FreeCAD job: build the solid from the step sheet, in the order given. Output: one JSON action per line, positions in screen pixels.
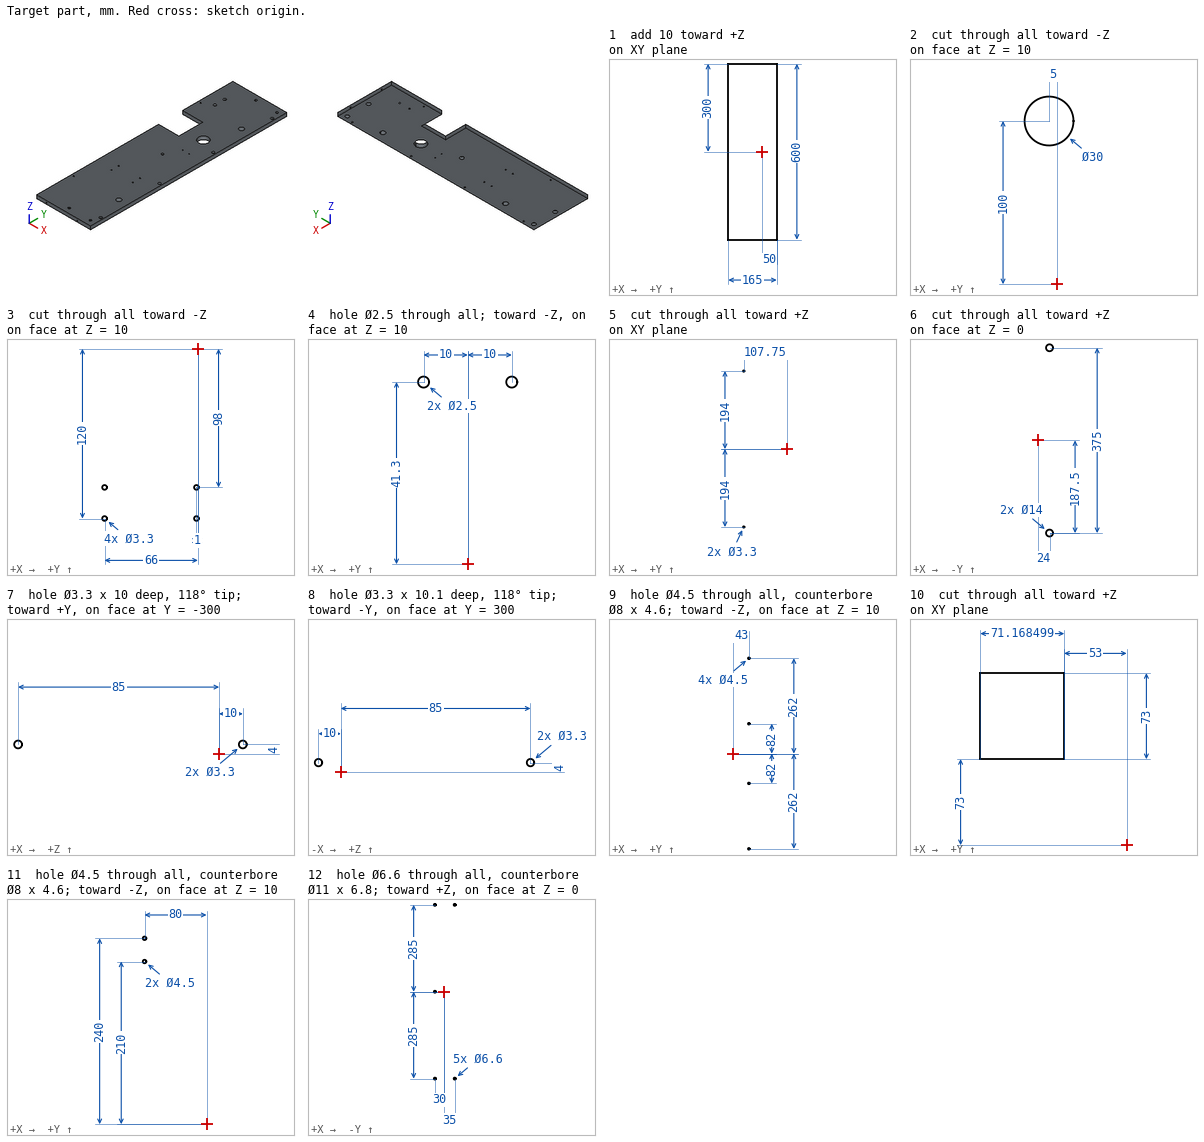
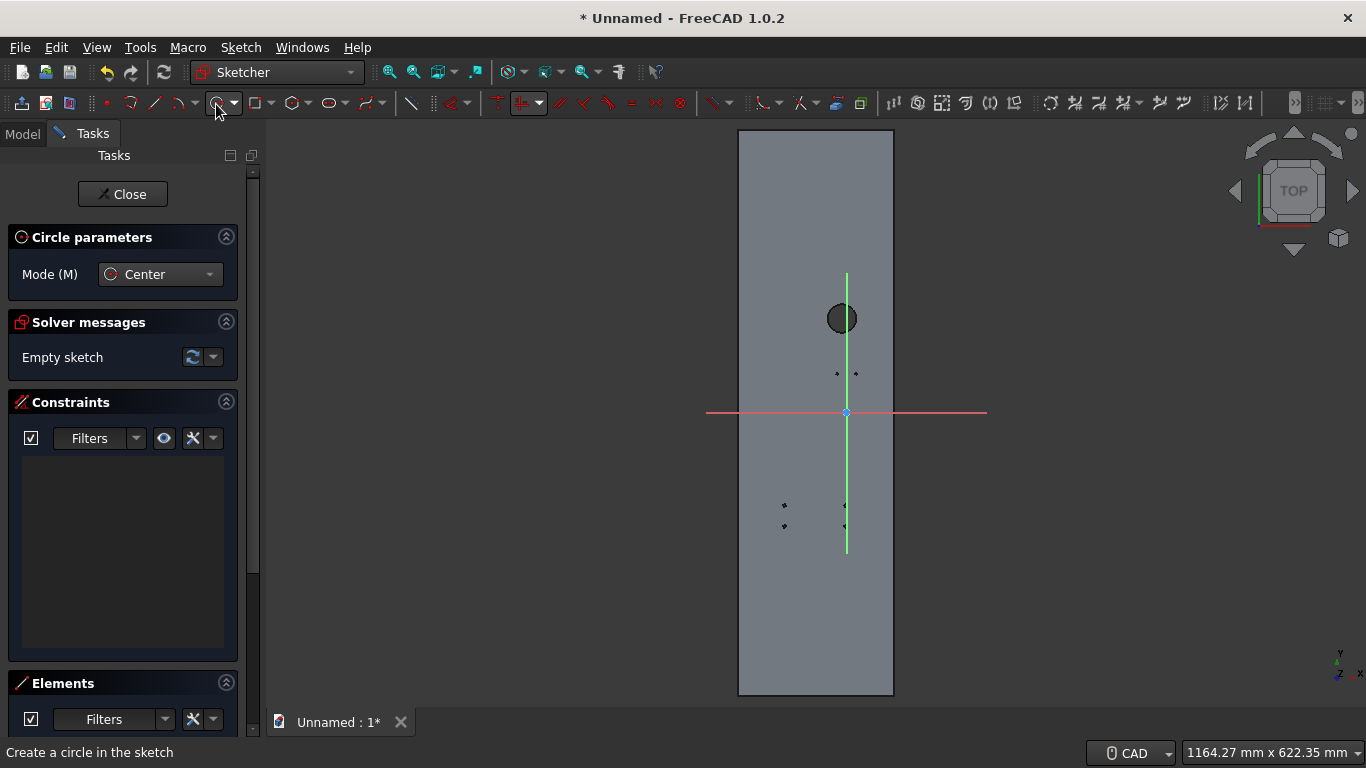
{"action": "scroll", "coordinate": [745, 230], "scroll_direction": "up", "scroll_amount": 14}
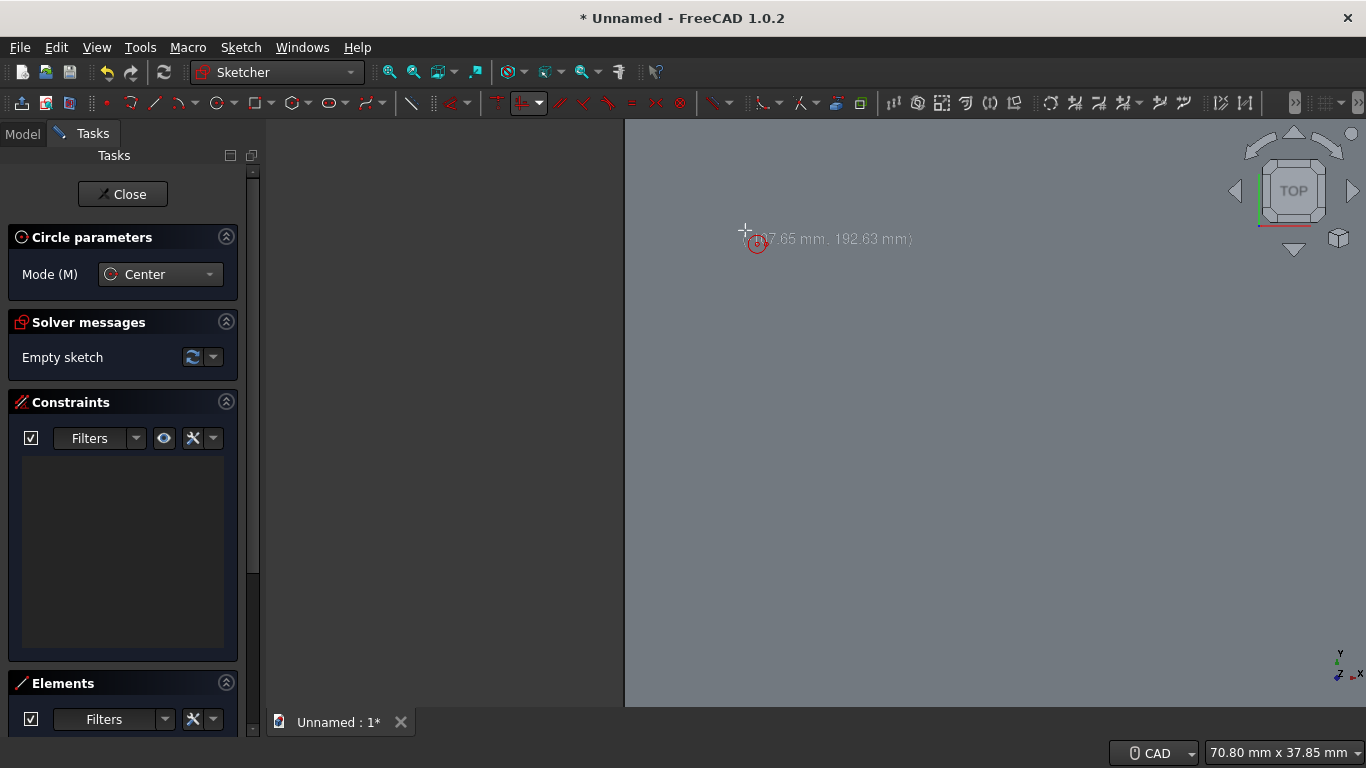
{"action": "scroll", "coordinate": [695, 230], "scroll_direction": "down", "scroll_amount": 14}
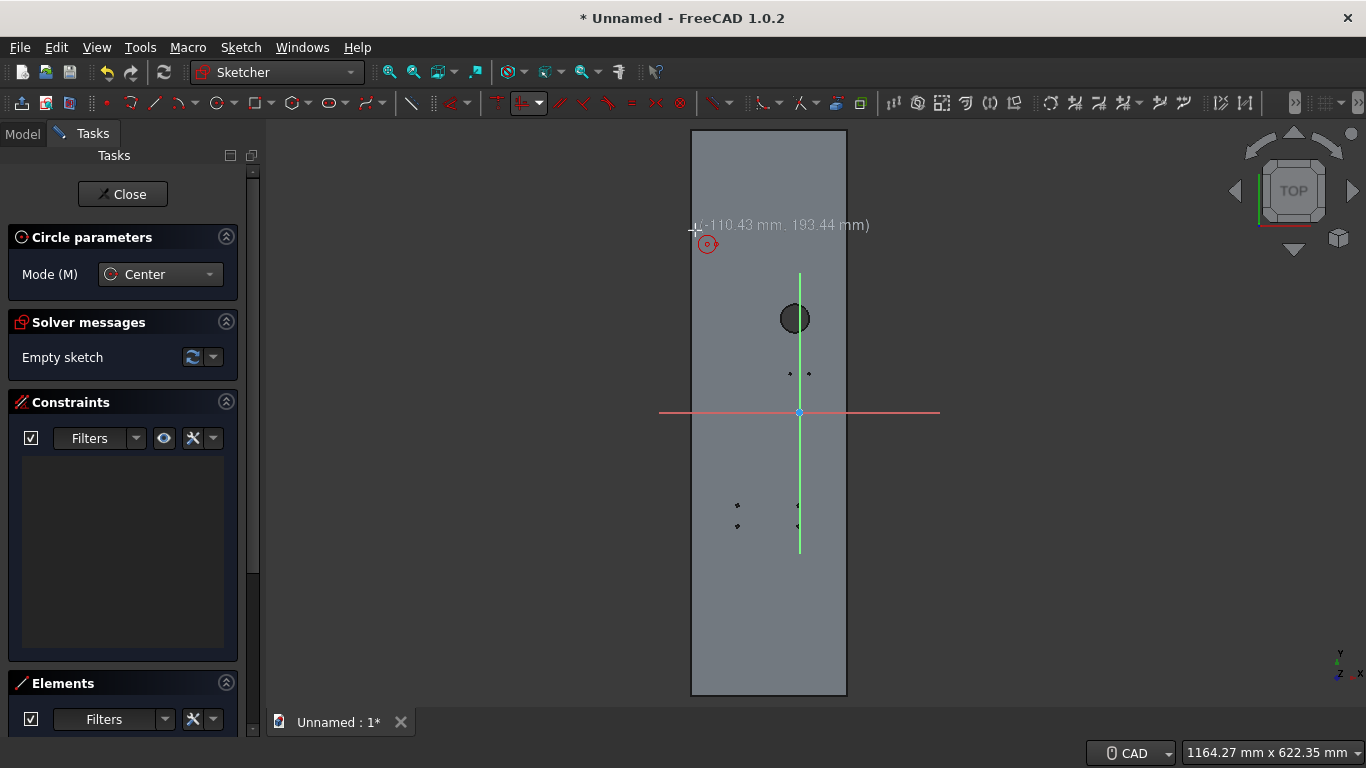
{"action": "left_click", "coordinate": [698, 230]}
{"action": "mouse_move", "coordinate": [699, 229]}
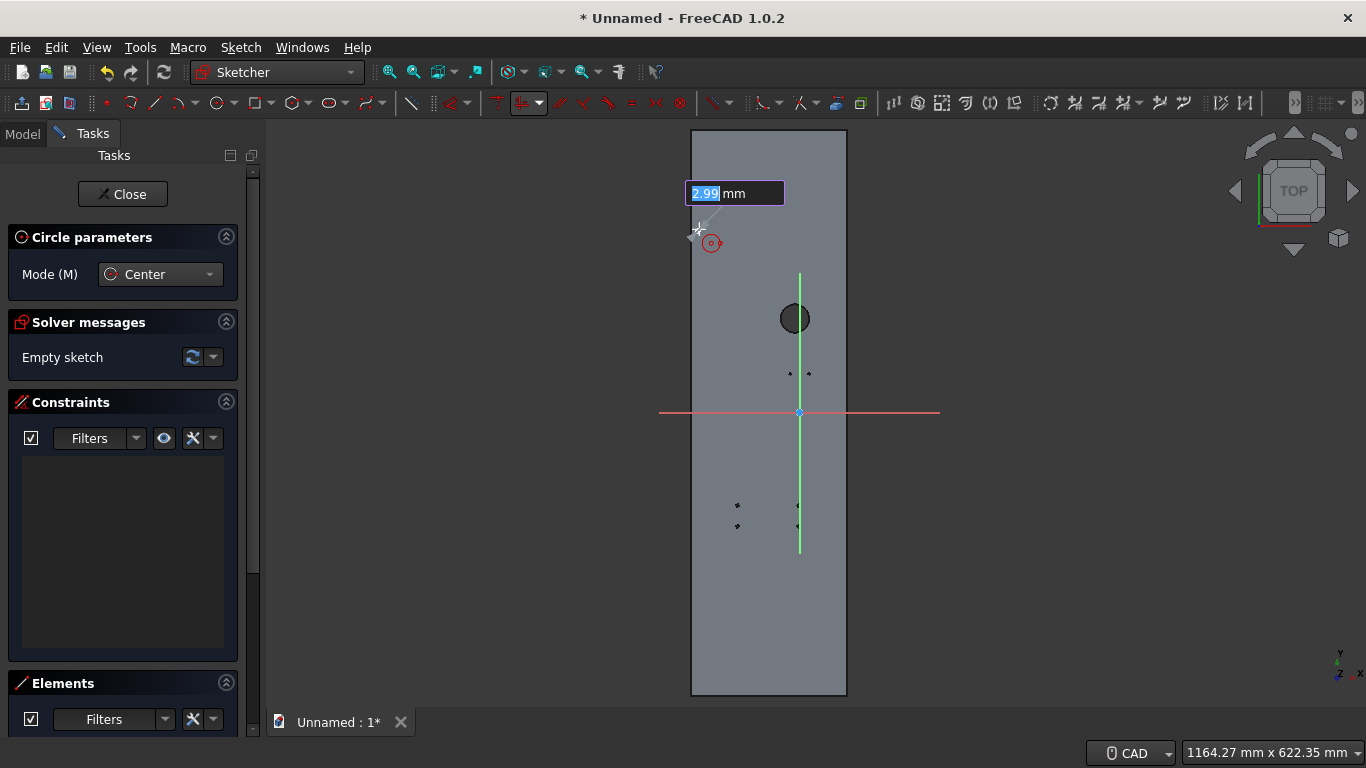
{"action": "type", "text": "3.3"}
{"action": "key", "text": "Return"}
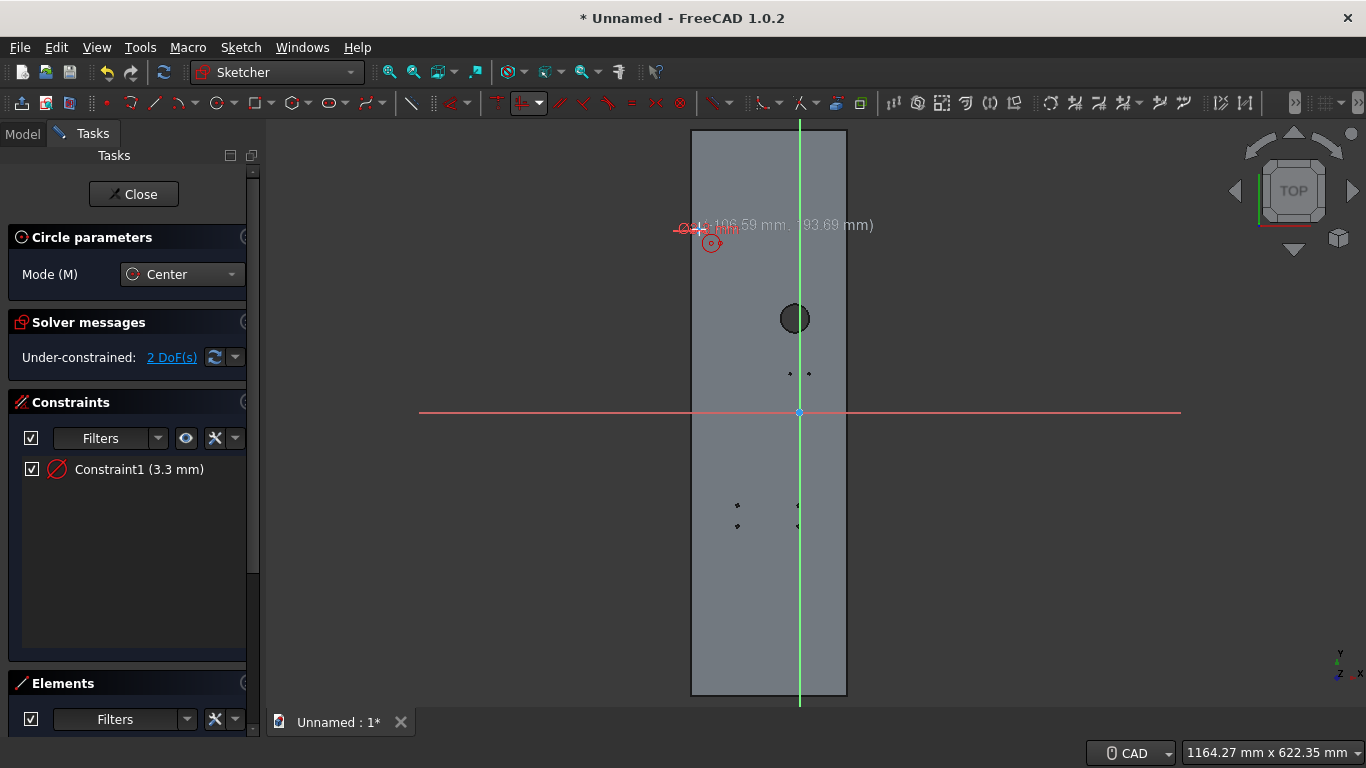
{"action": "scroll", "coordinate": [698, 596], "scroll_direction": "up", "scroll_amount": 14}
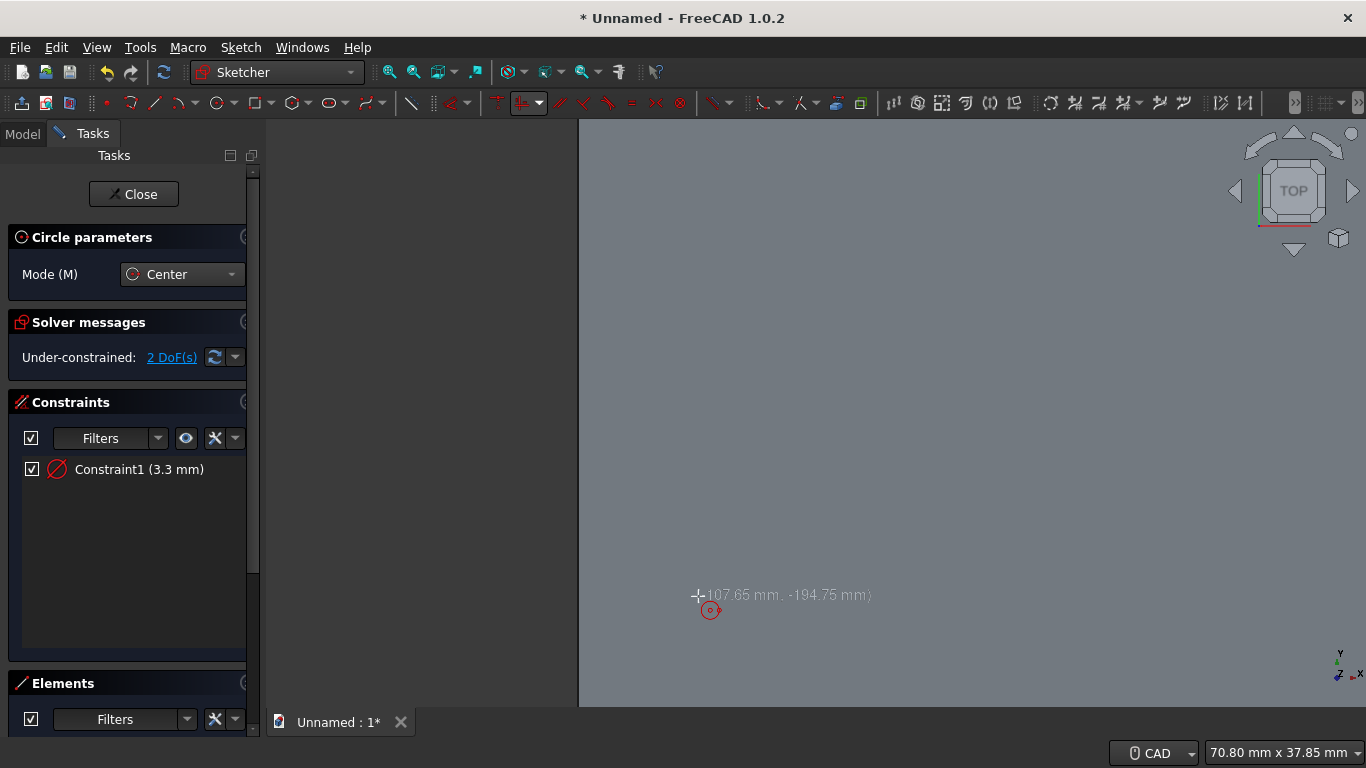
{"action": "scroll", "coordinate": [698, 597], "scroll_direction": "down", "scroll_amount": 14}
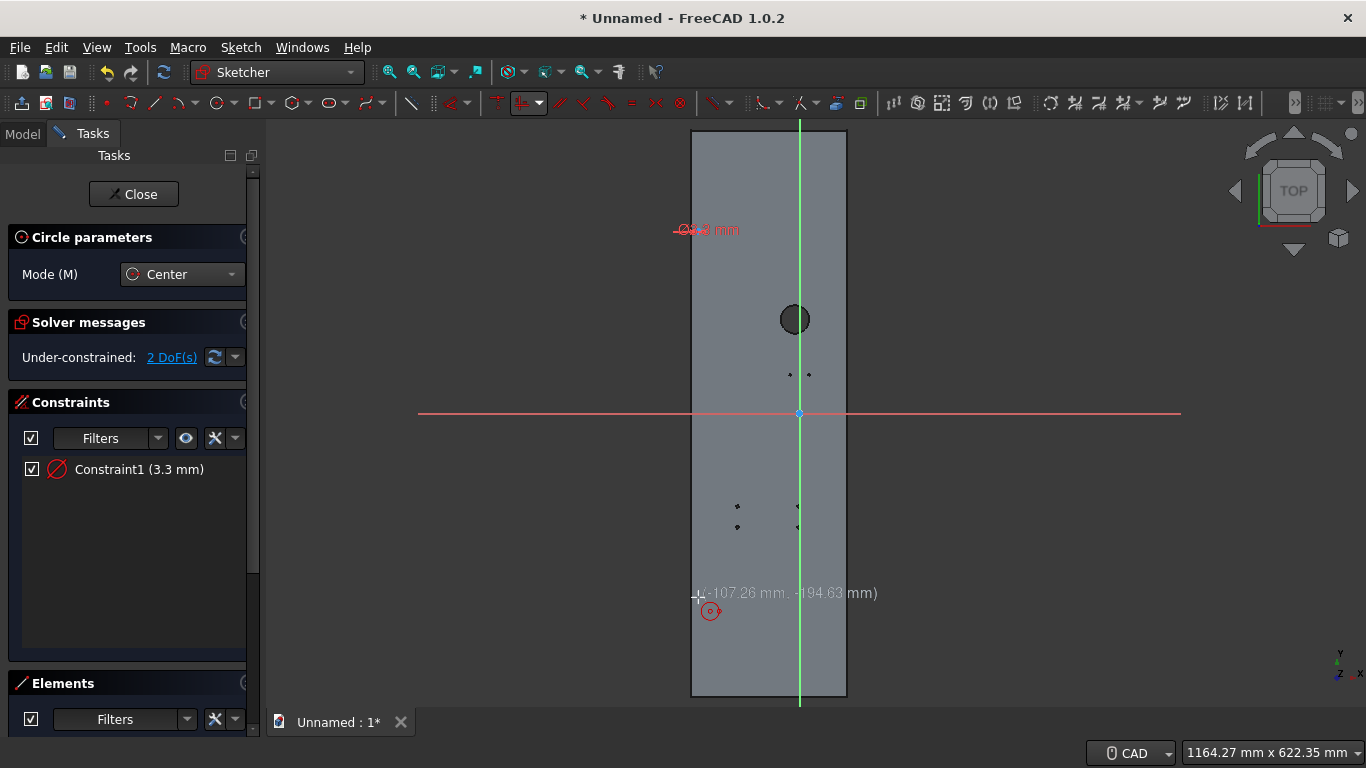
{"action": "left_click", "coordinate": [698, 597]}
{"action": "mouse_move", "coordinate": [699, 596]}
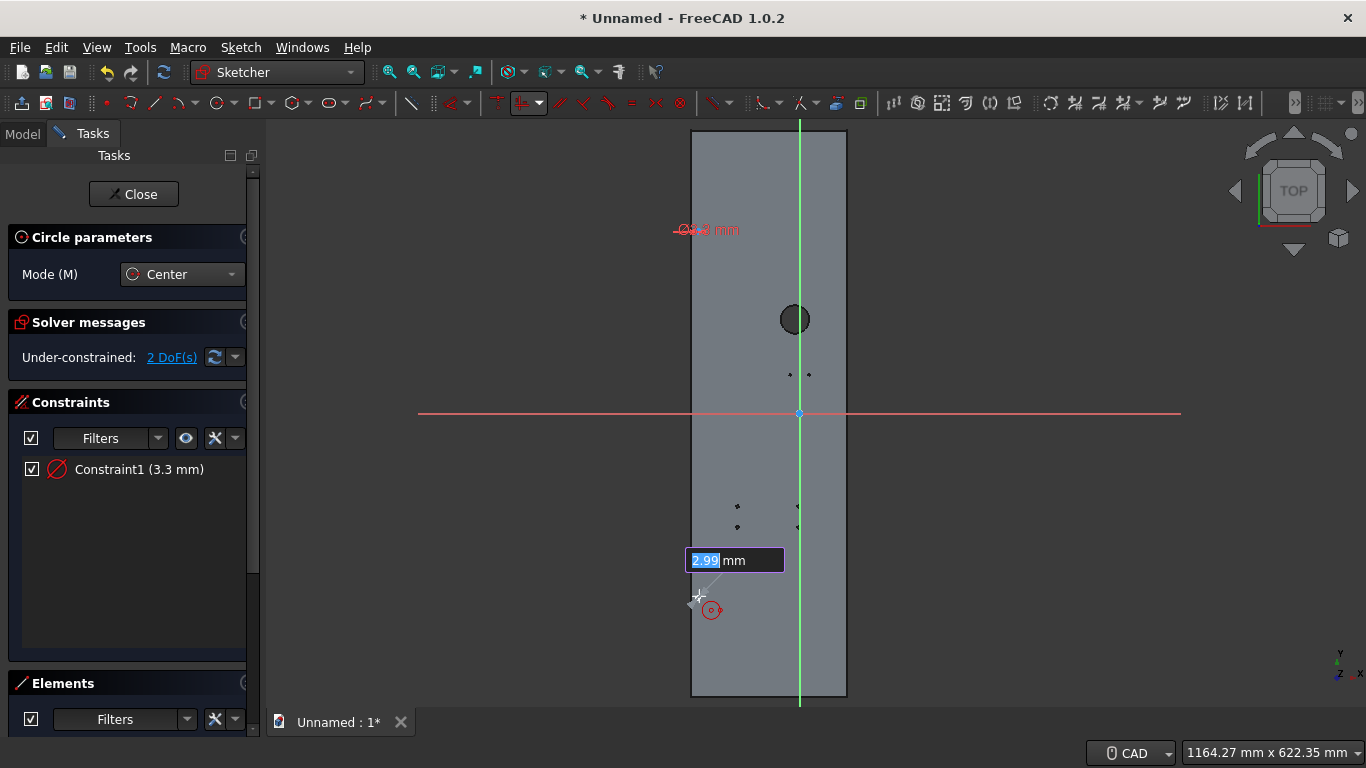
{"action": "type", "text": "3.3"}
{"action": "key", "text": "Return"}
{"action": "key", "text": "Escape"}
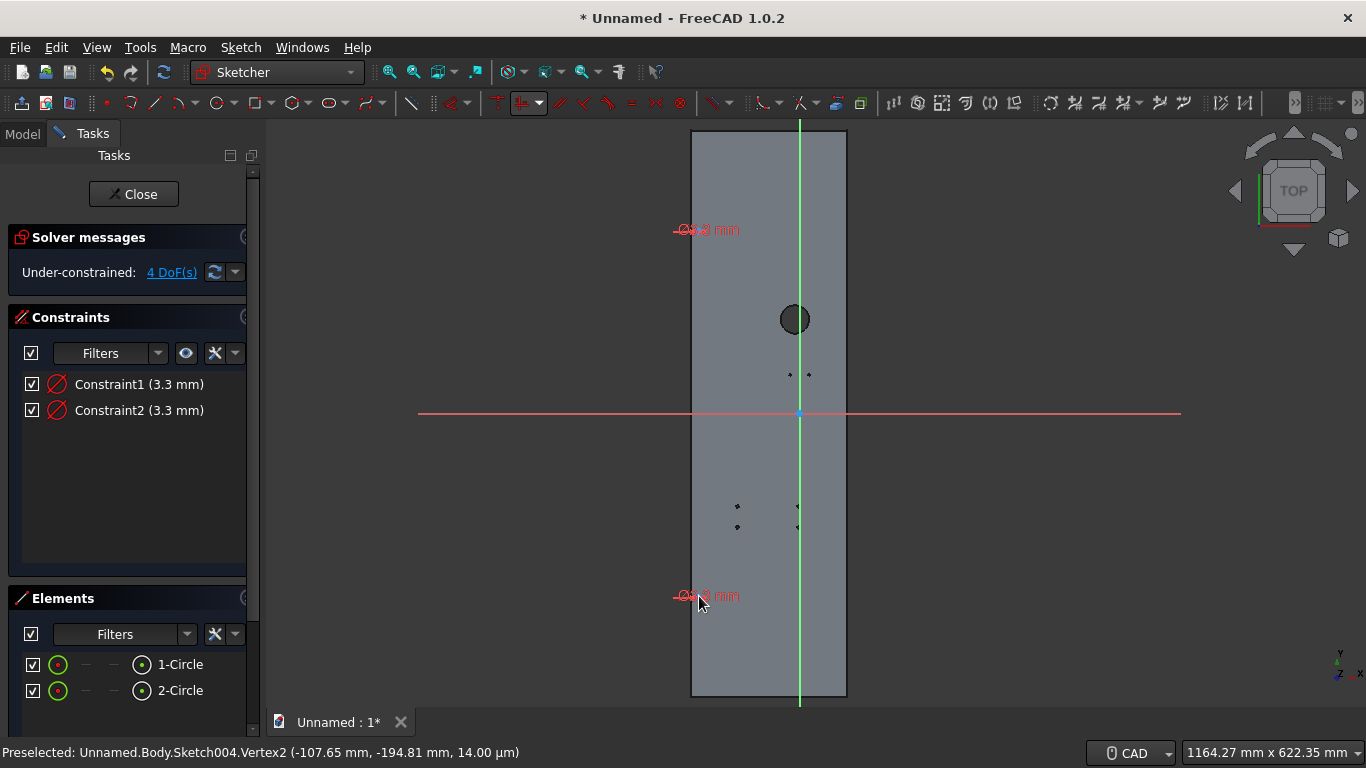
{"action": "left_click", "coordinate": [698, 232]}